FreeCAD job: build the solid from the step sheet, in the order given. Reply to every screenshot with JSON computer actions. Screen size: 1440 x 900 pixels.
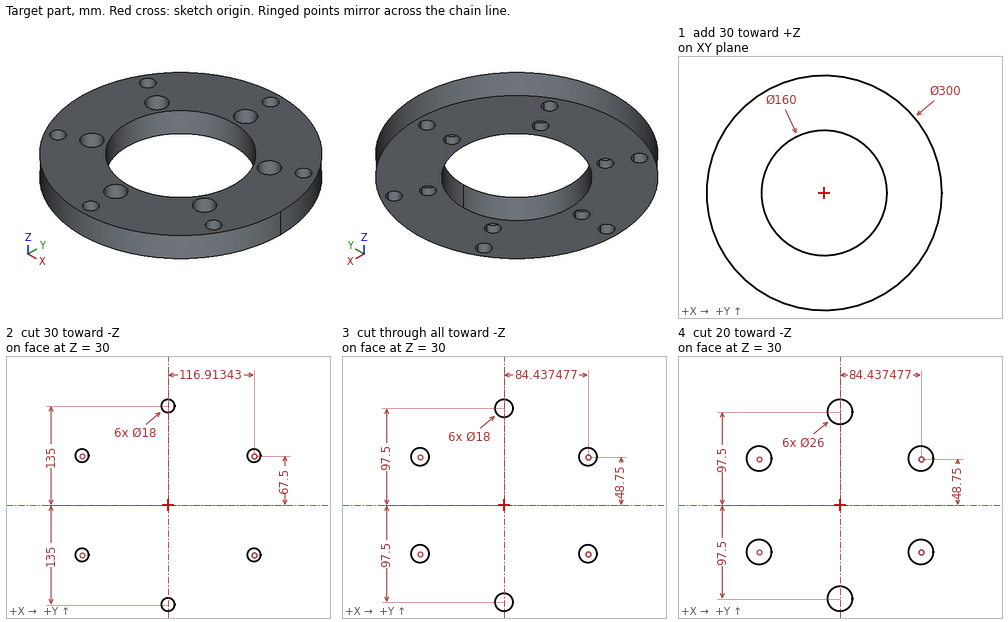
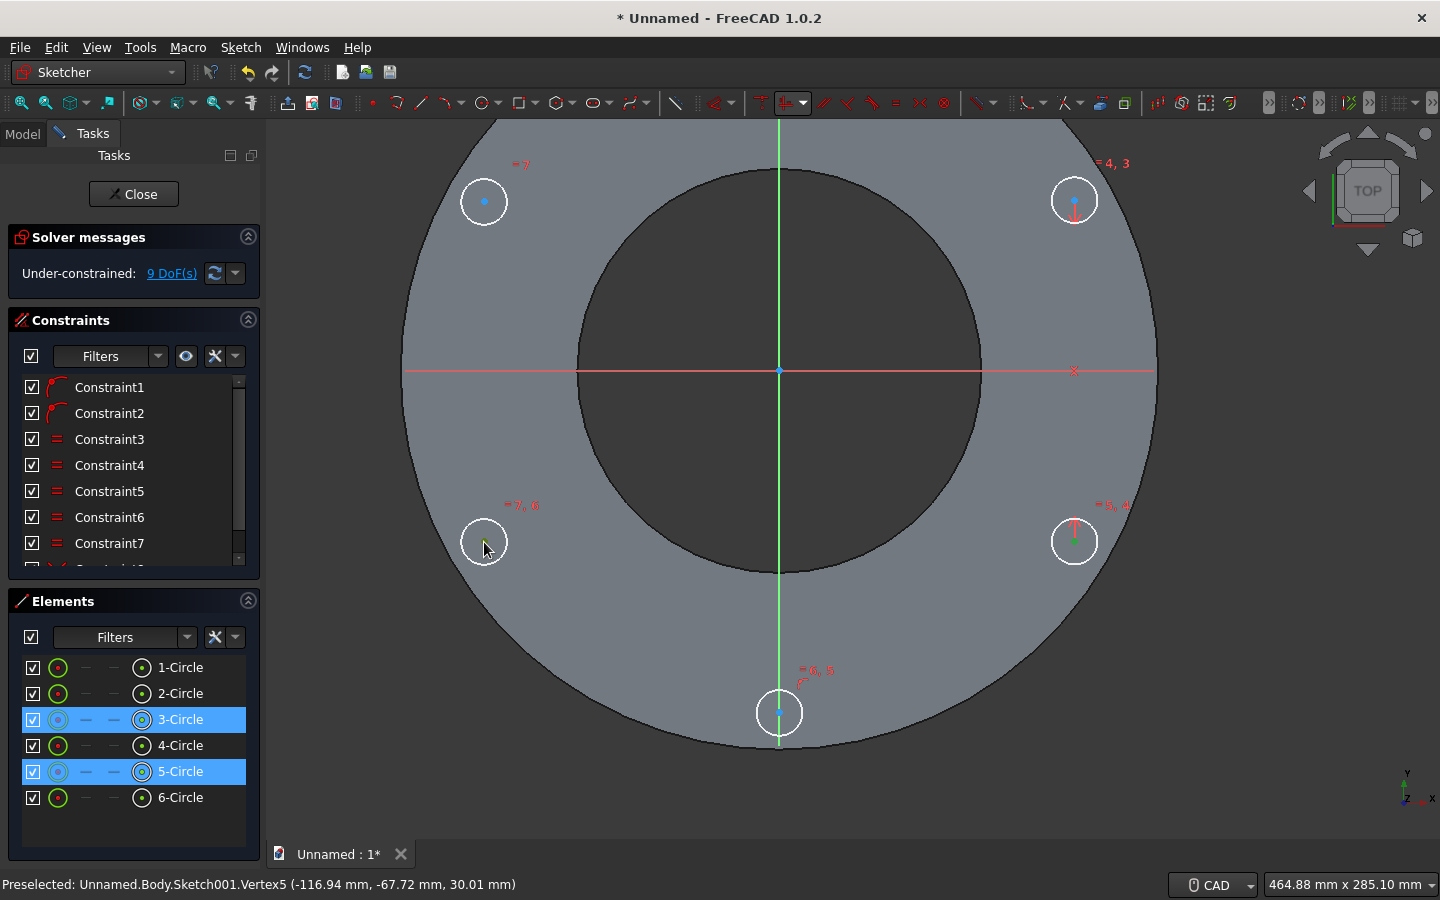
{"action": "left_click", "coordinate": [779, 621]}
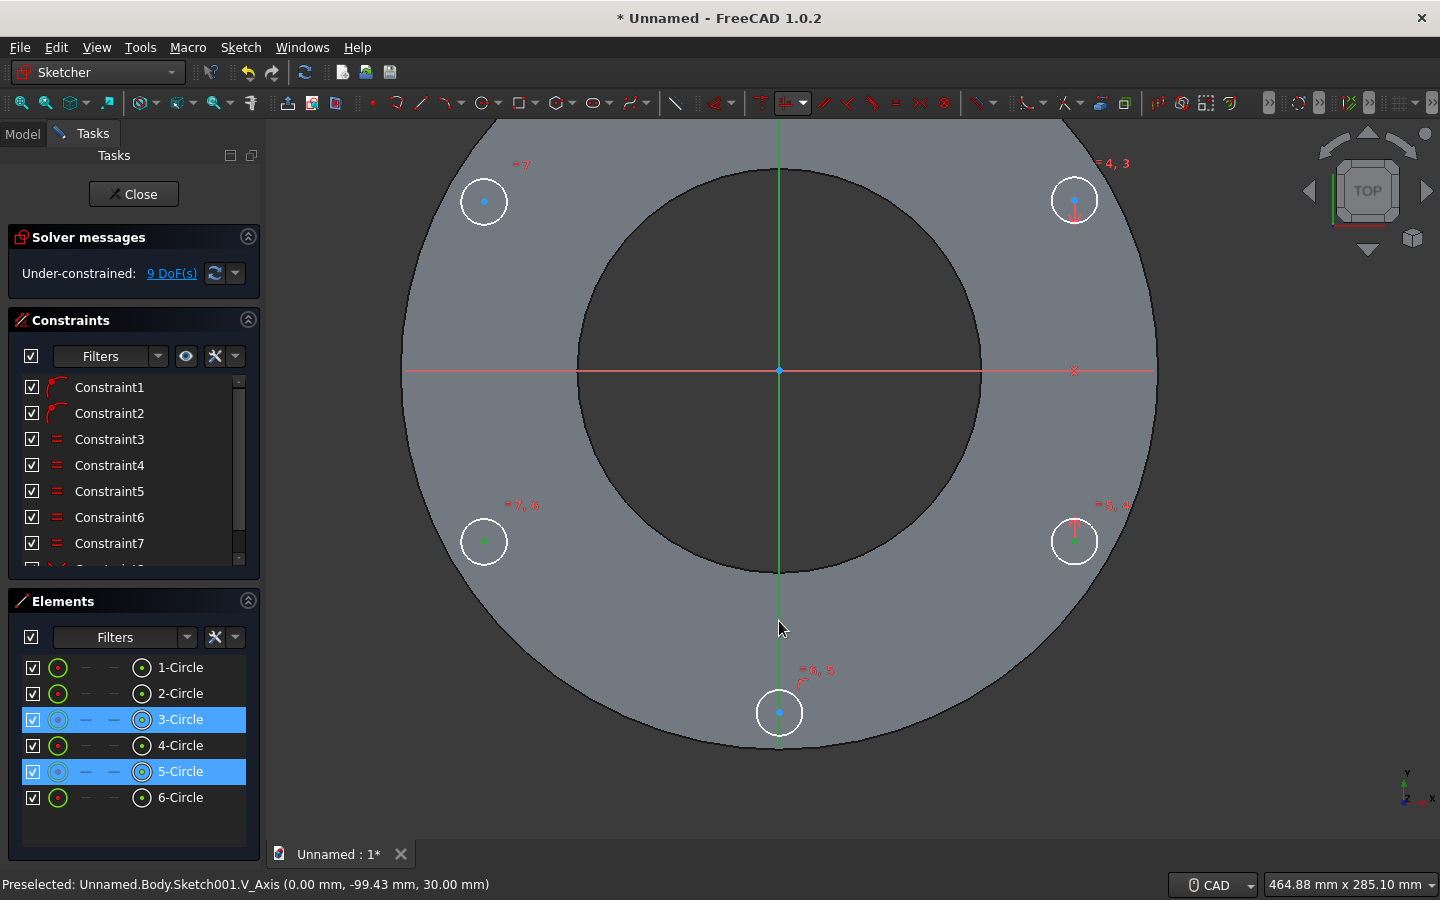
{"action": "key", "text": "s"}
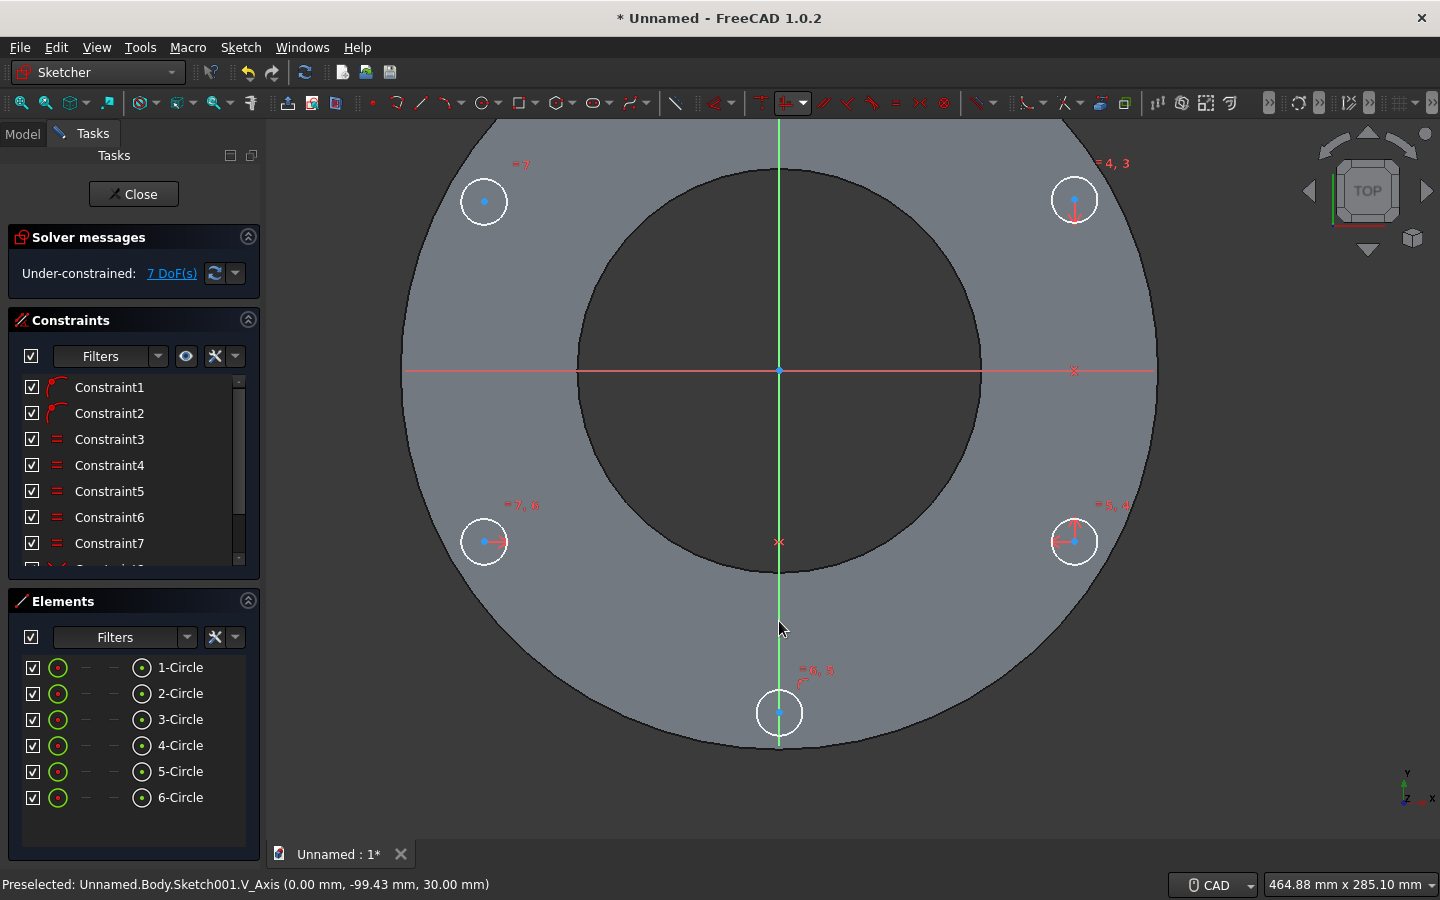
{"action": "left_click", "coordinate": [1075, 200]}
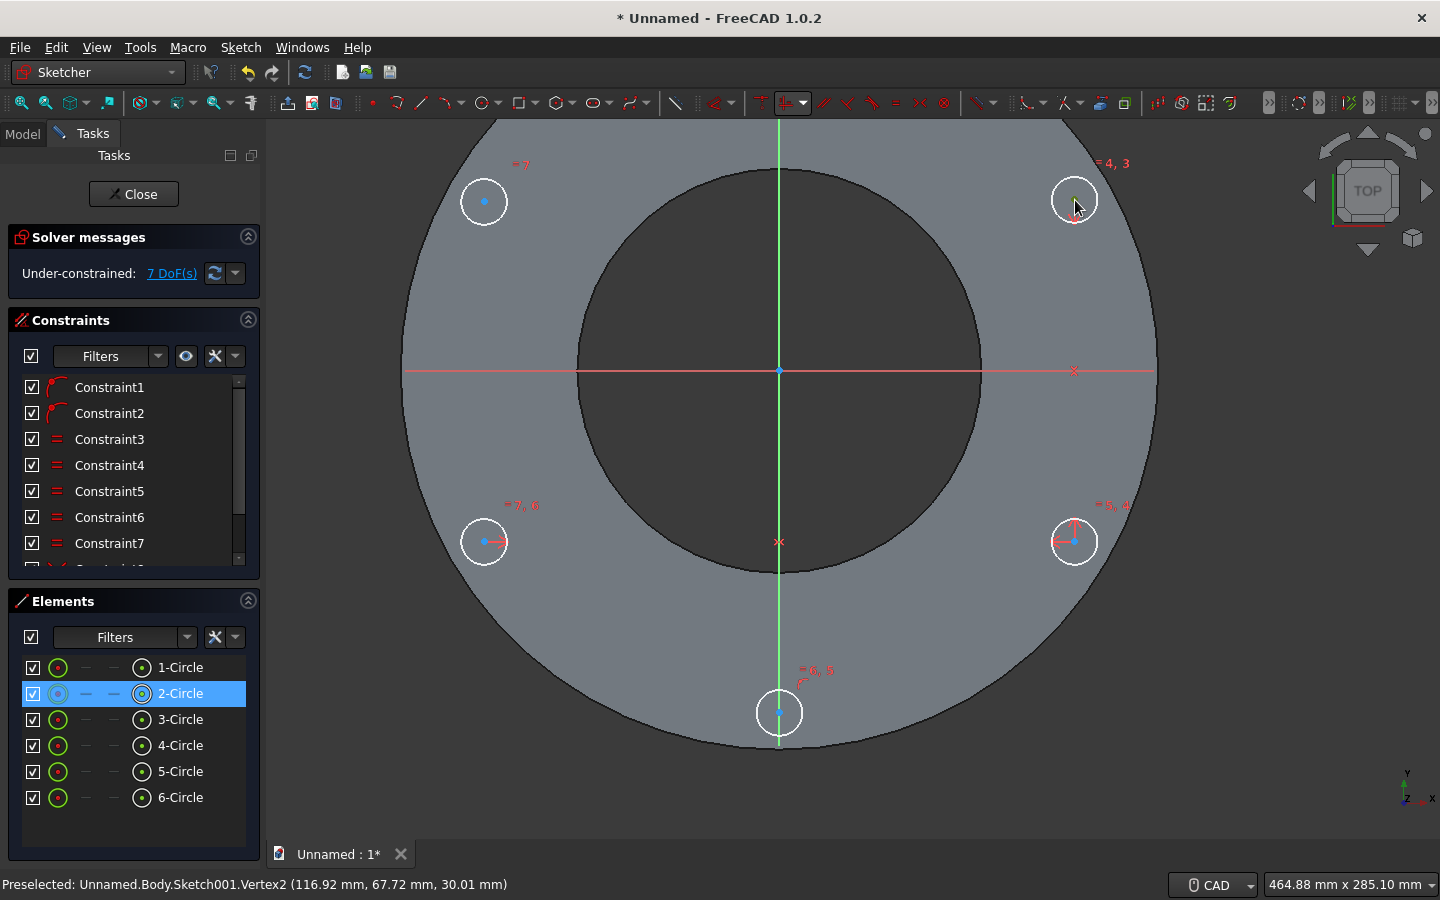
{"action": "left_click", "coordinate": [484, 202]}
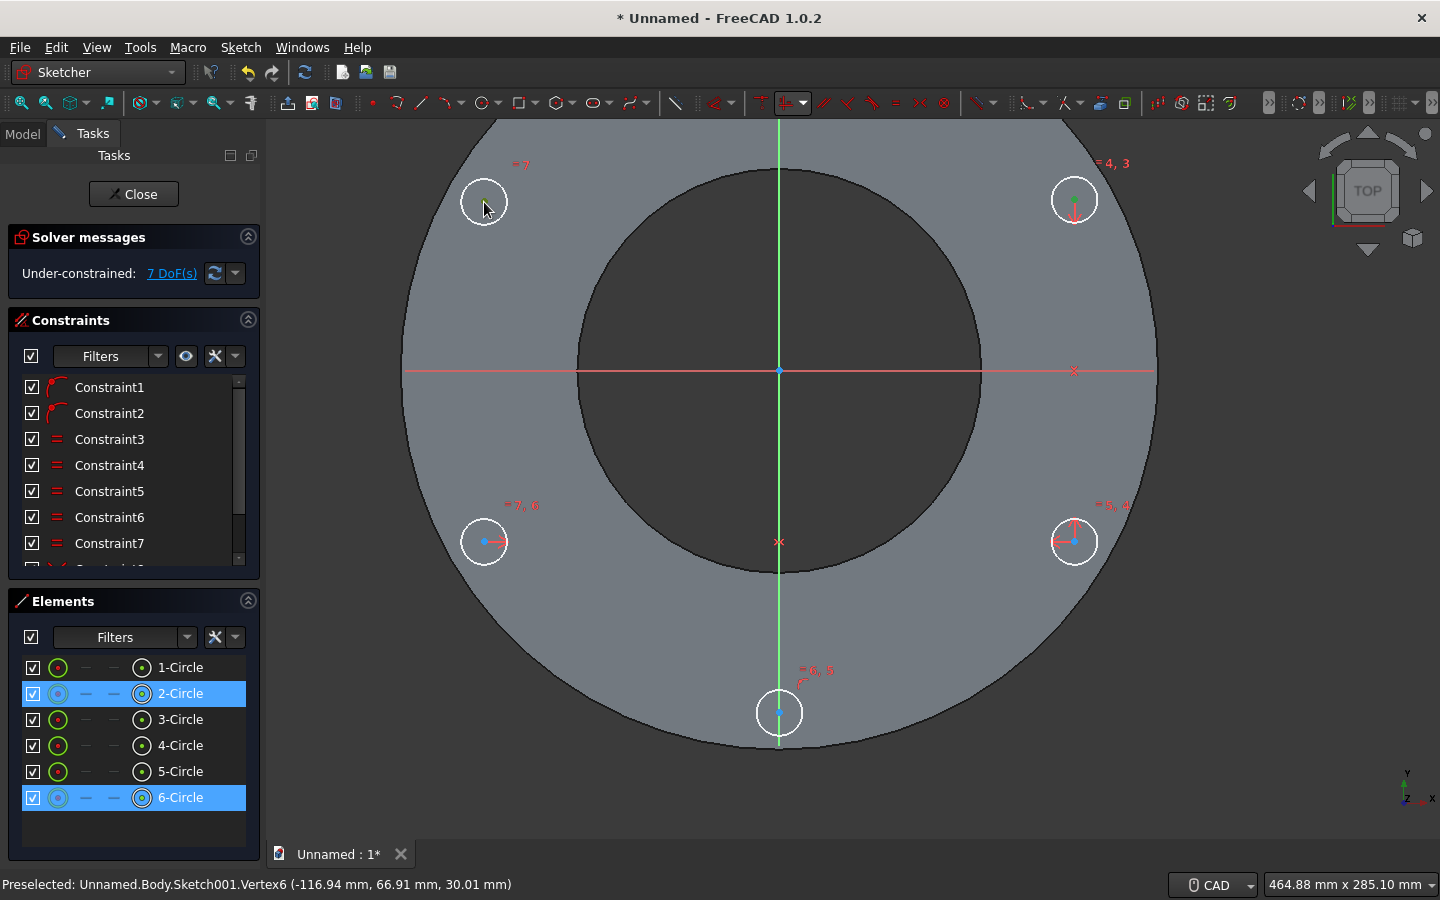
{"action": "left_click", "coordinate": [779, 621]}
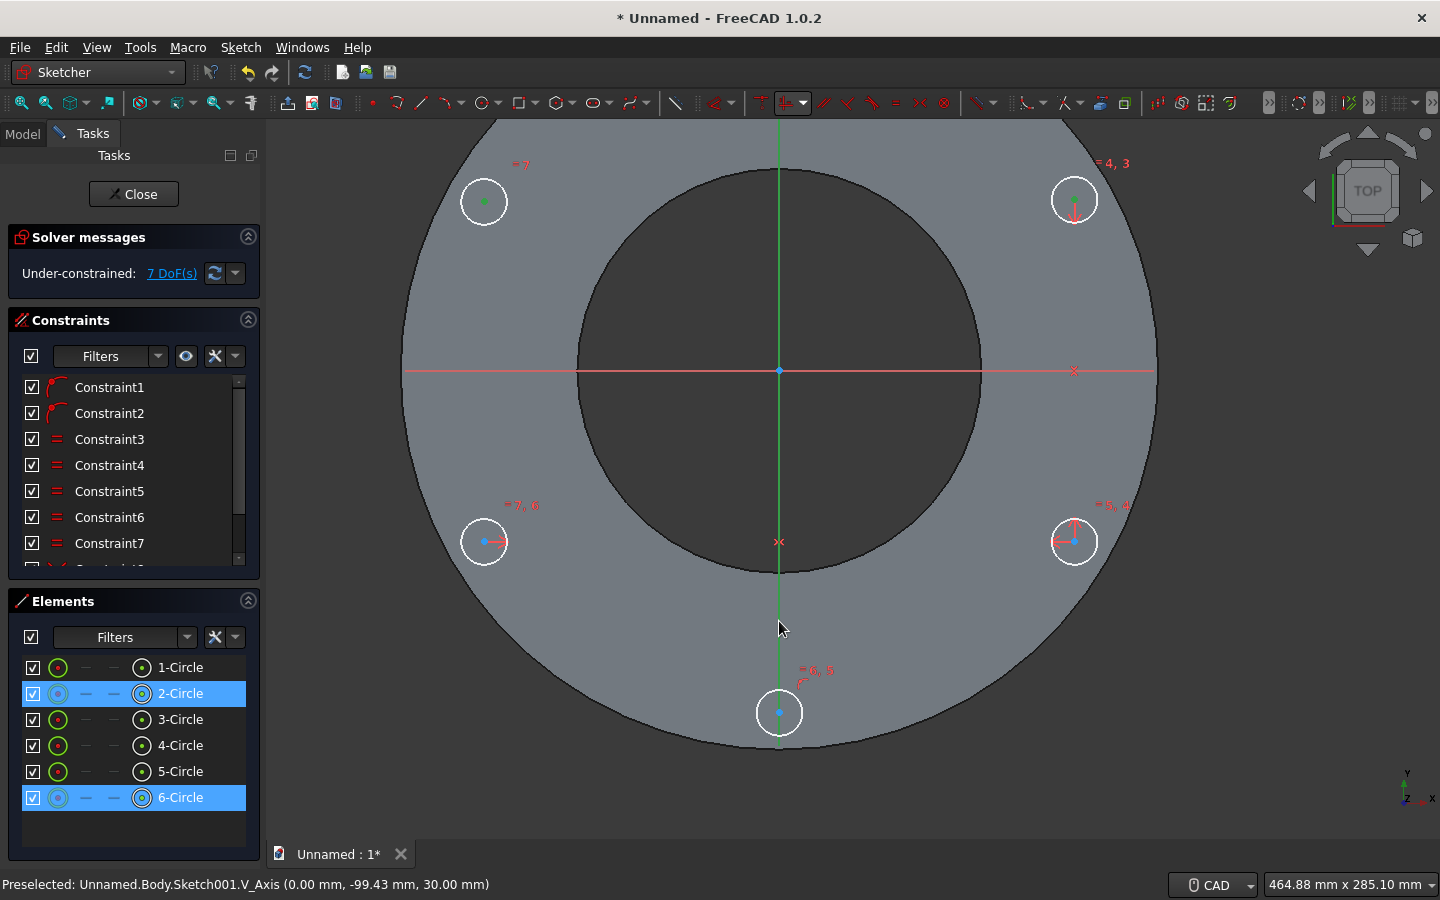
{"action": "key", "text": "s"}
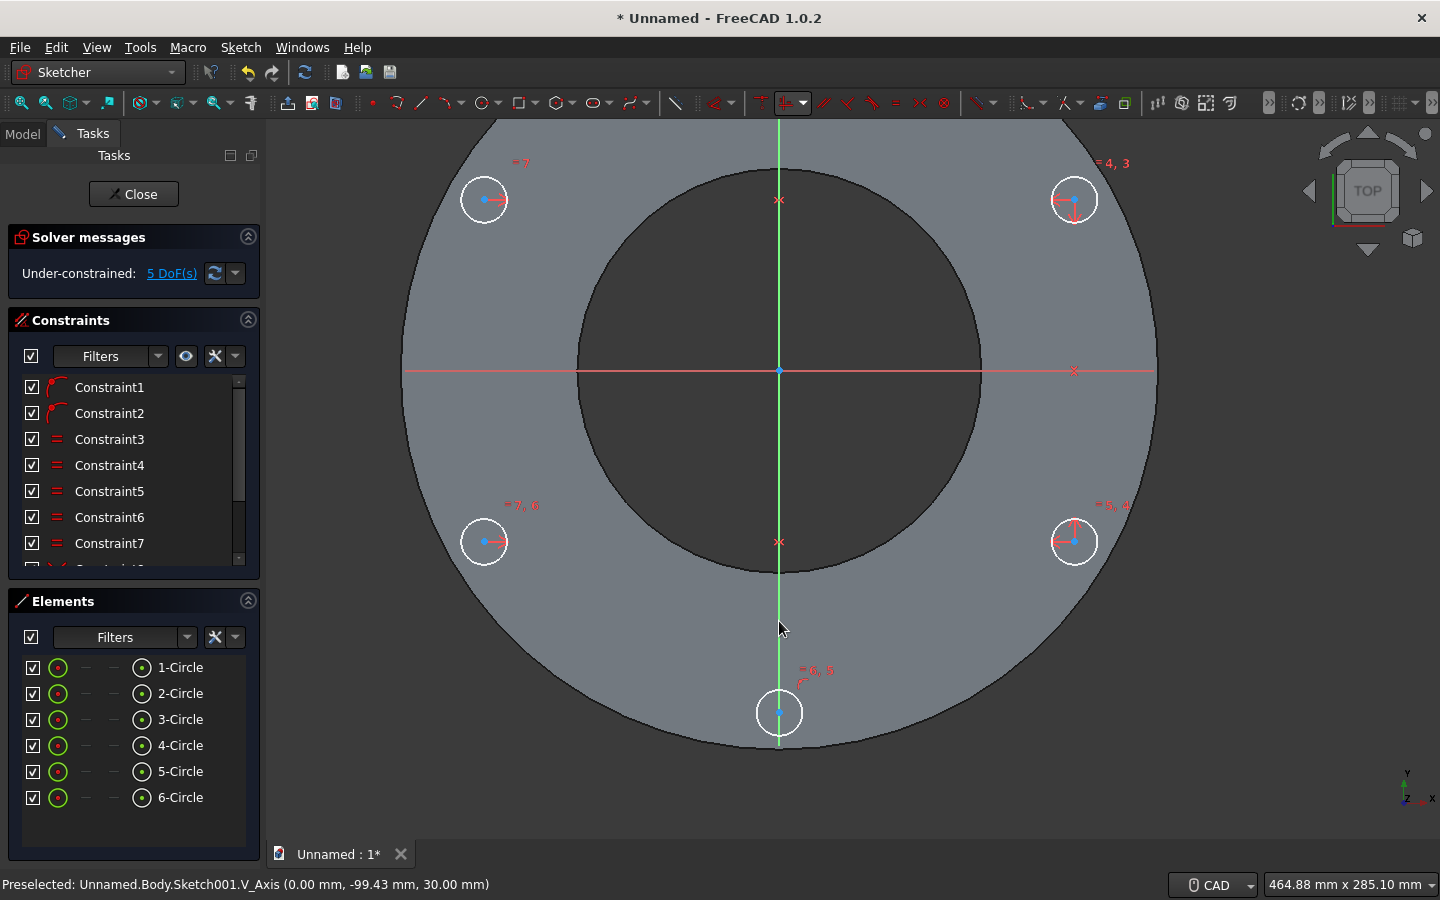
{"action": "scroll", "coordinate": [795, 699], "scroll_direction": "down", "scroll_amount": 2}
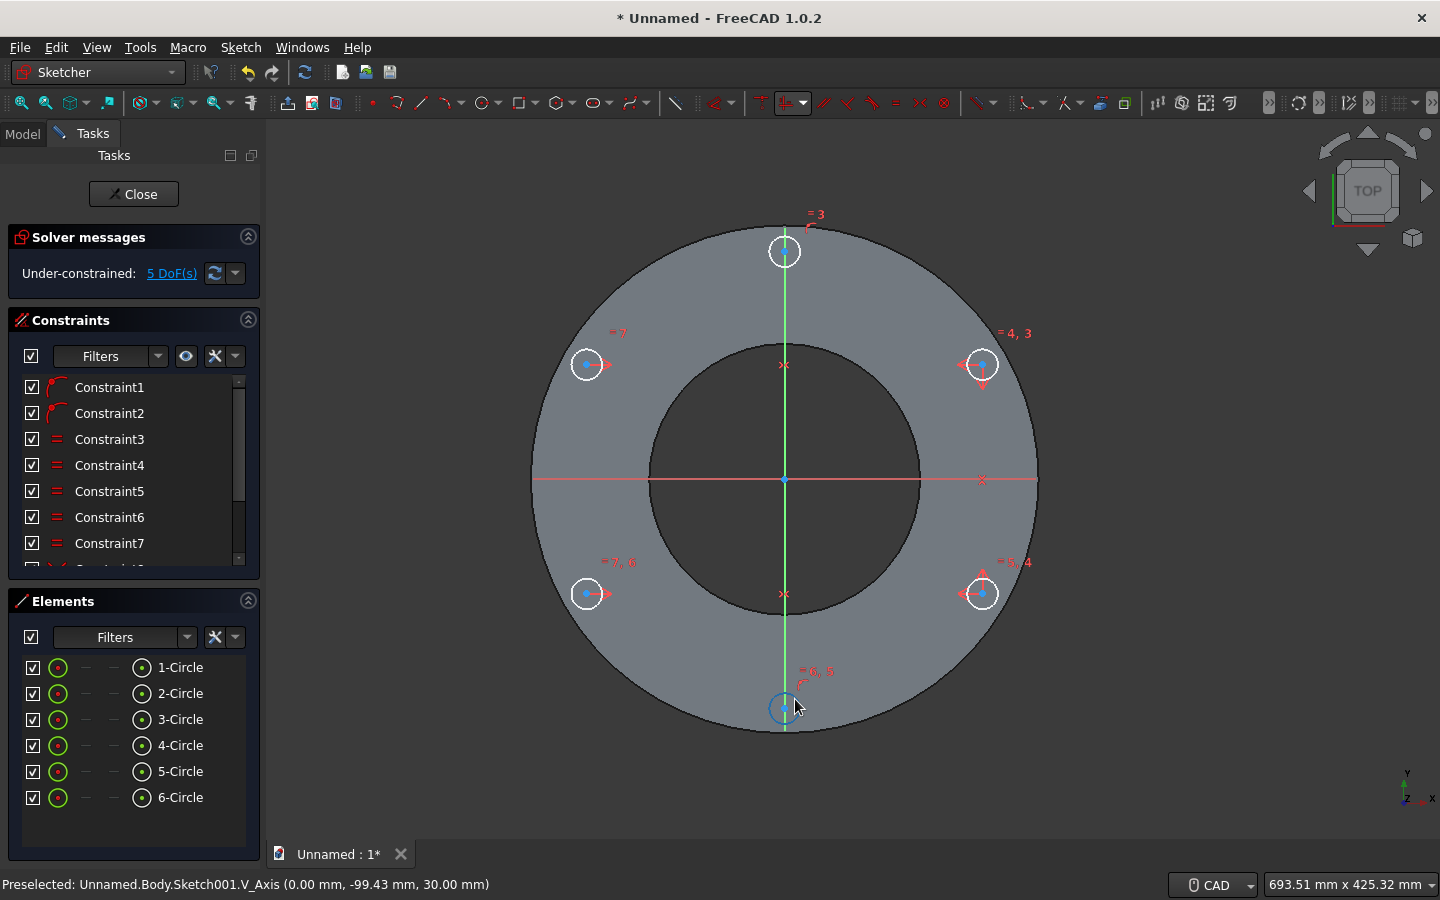
{"action": "scroll", "coordinate": [795, 241], "scroll_direction": "up", "scroll_amount": 2}